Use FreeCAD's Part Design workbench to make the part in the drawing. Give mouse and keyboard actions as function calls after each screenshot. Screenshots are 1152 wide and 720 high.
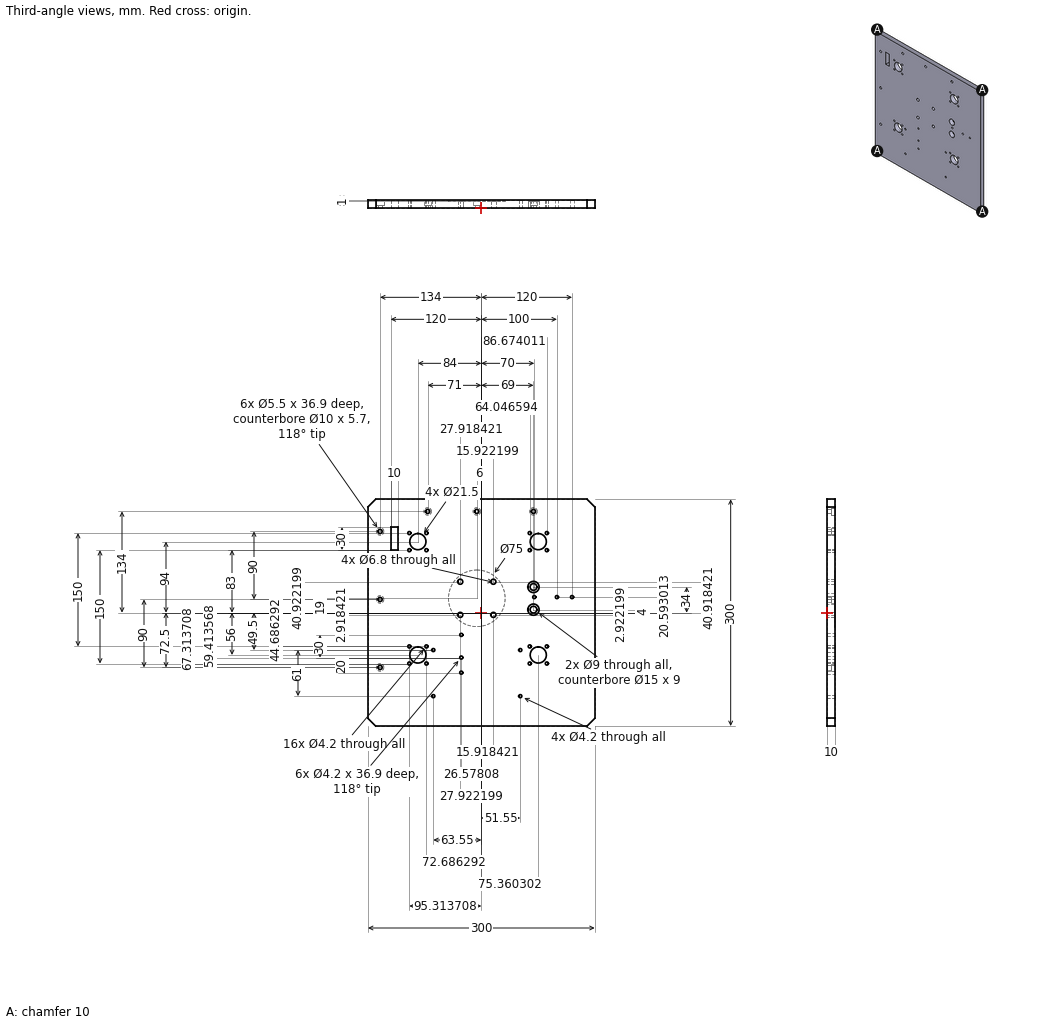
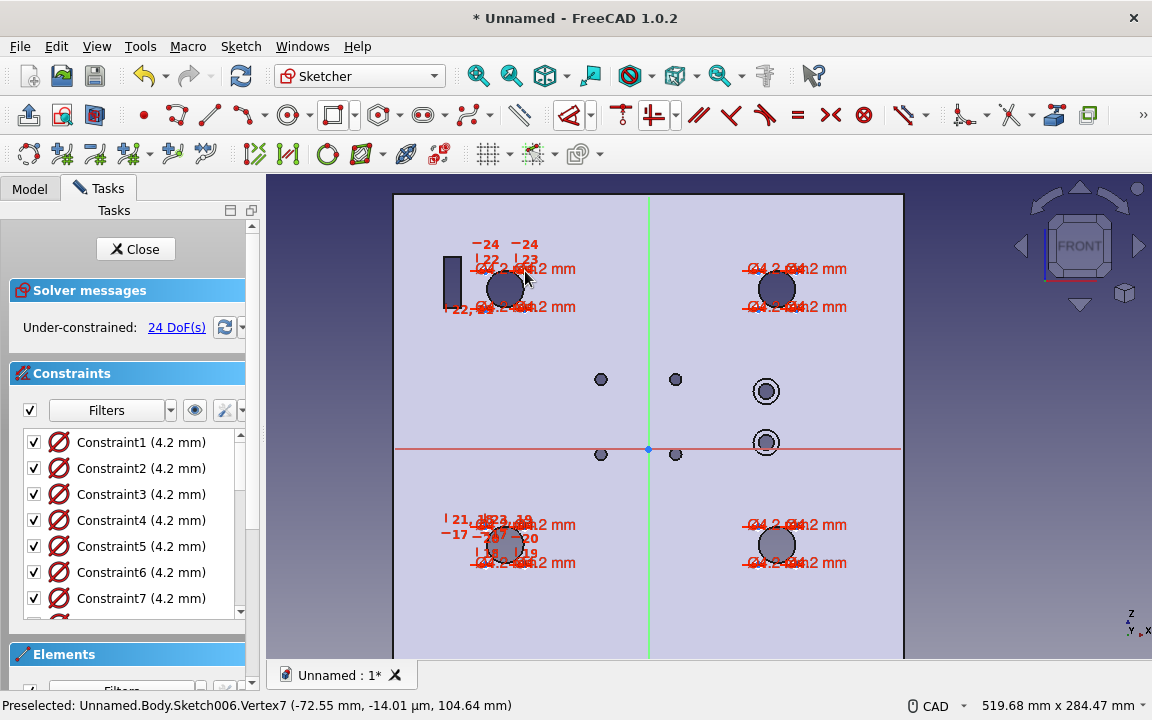
click(525, 309)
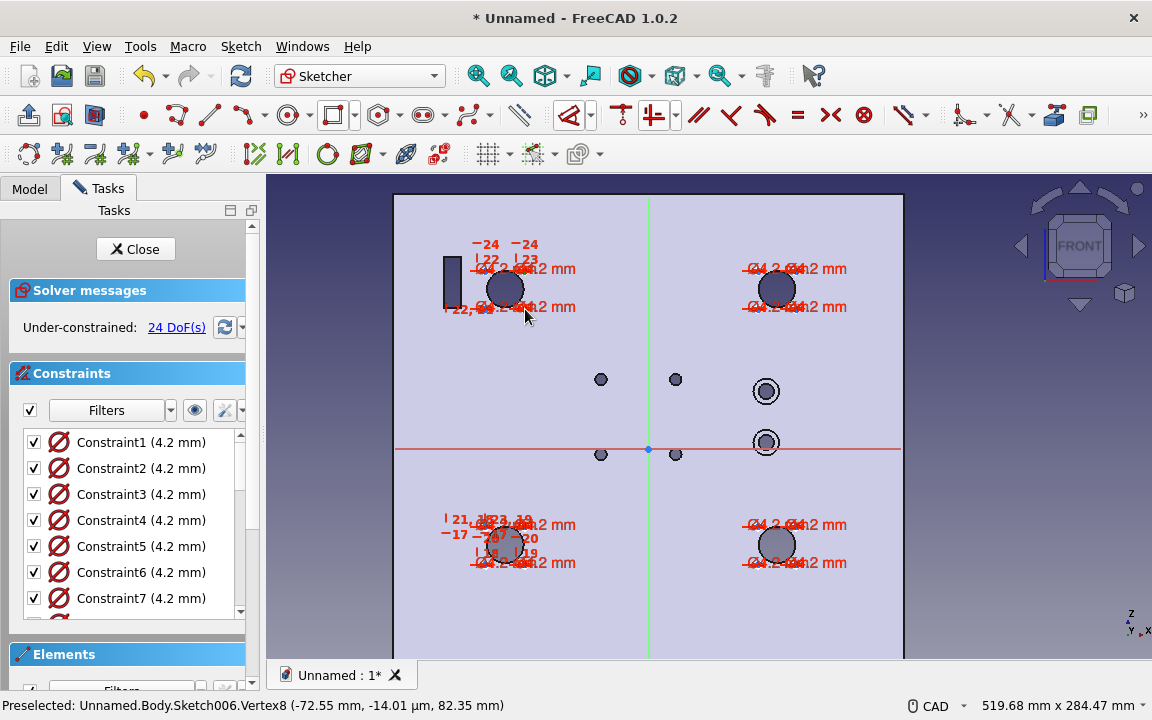
key(v)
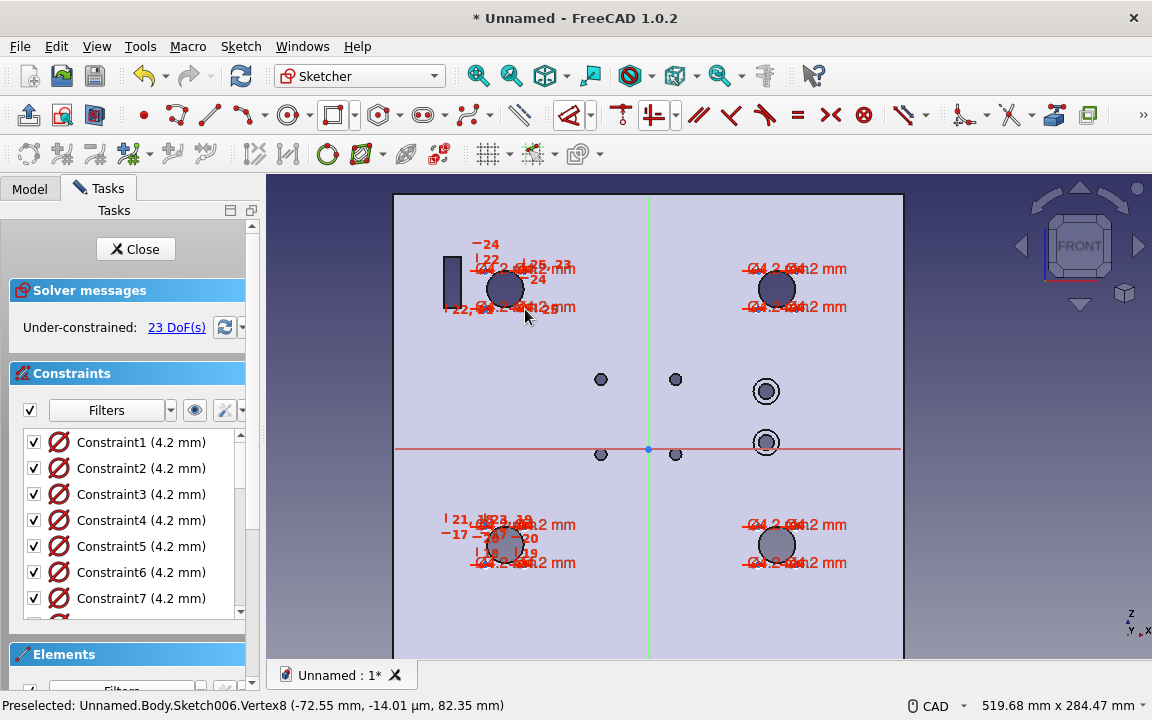
click(486, 309)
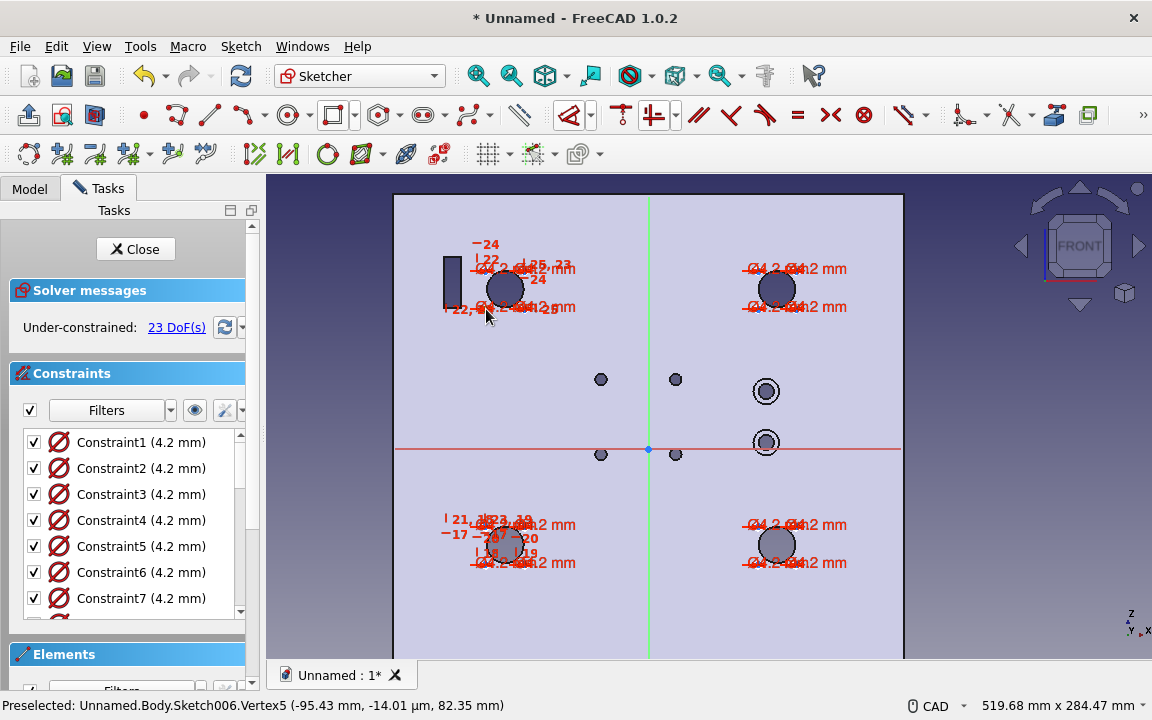
click(525, 309)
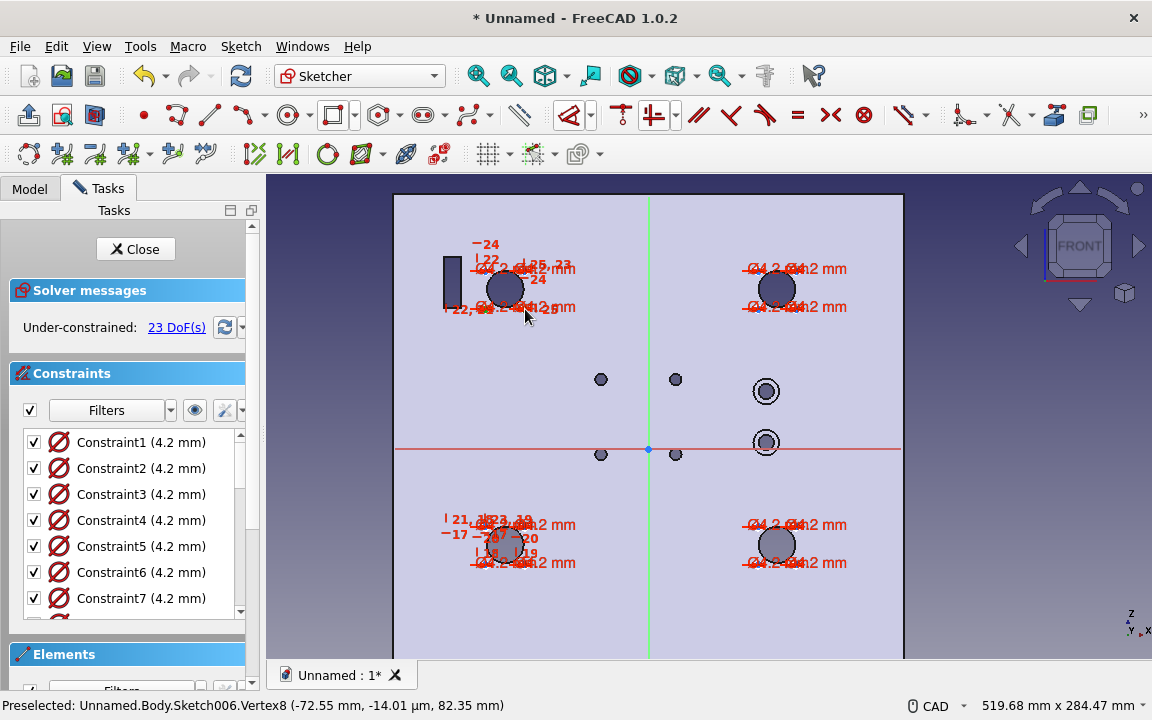
click(676, 116)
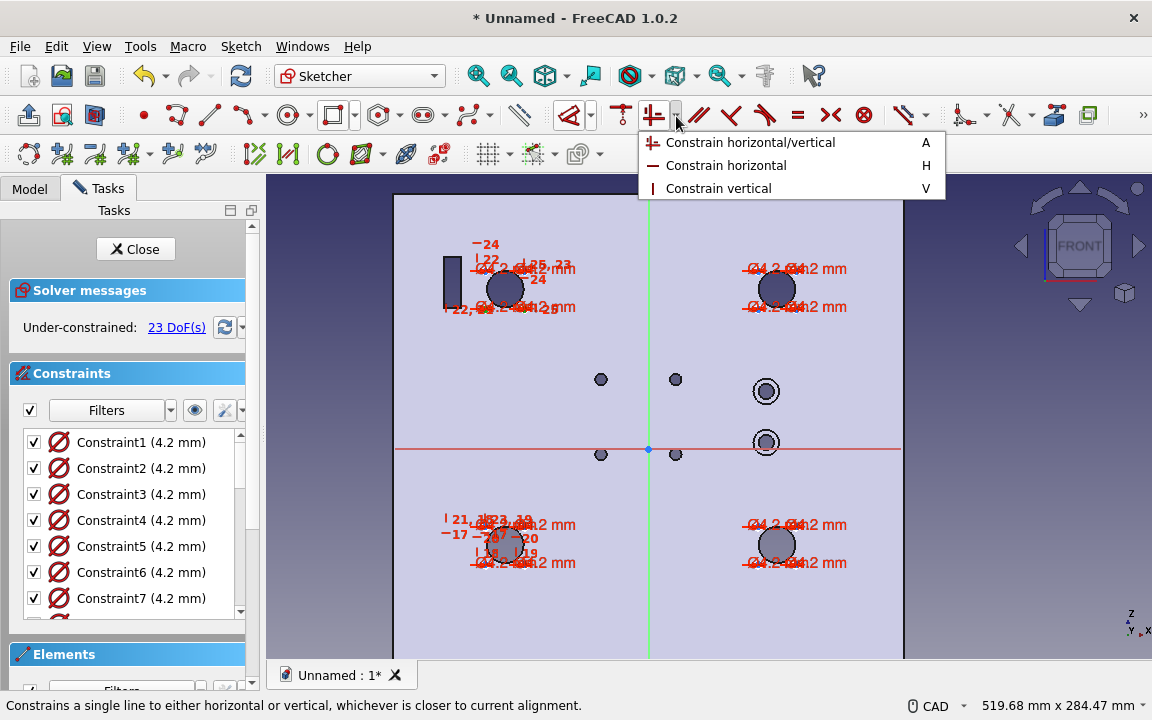
click(792, 166)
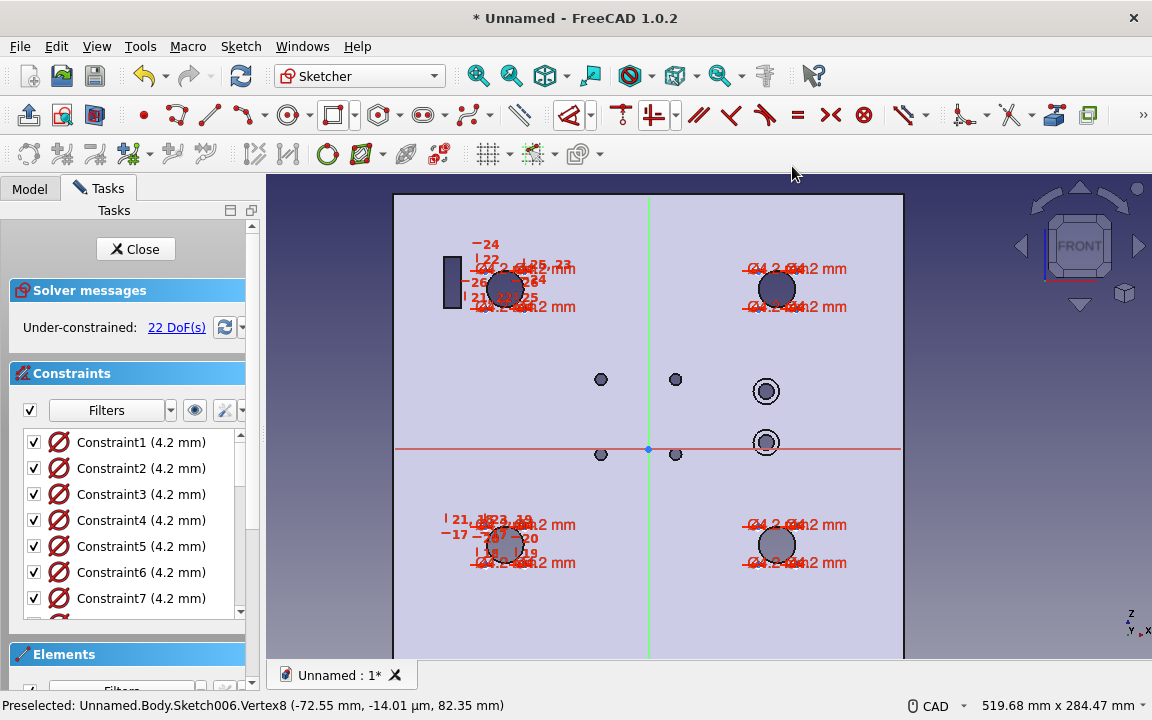
click(525, 309)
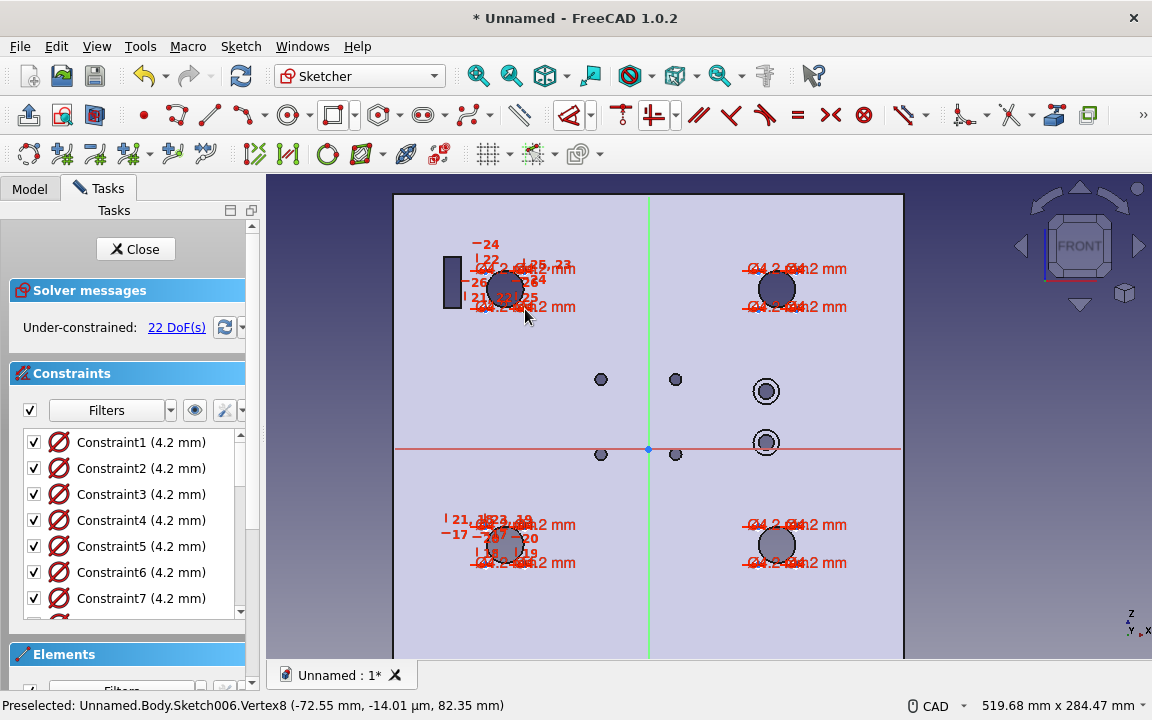
click(758, 309)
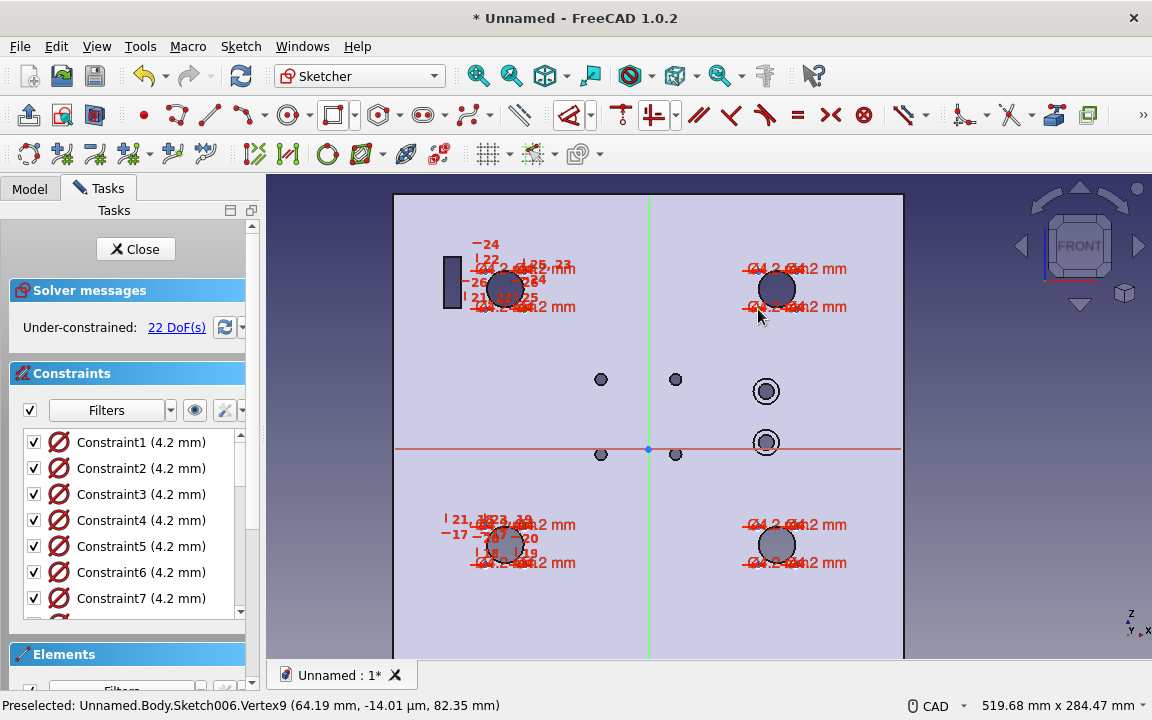
key(h)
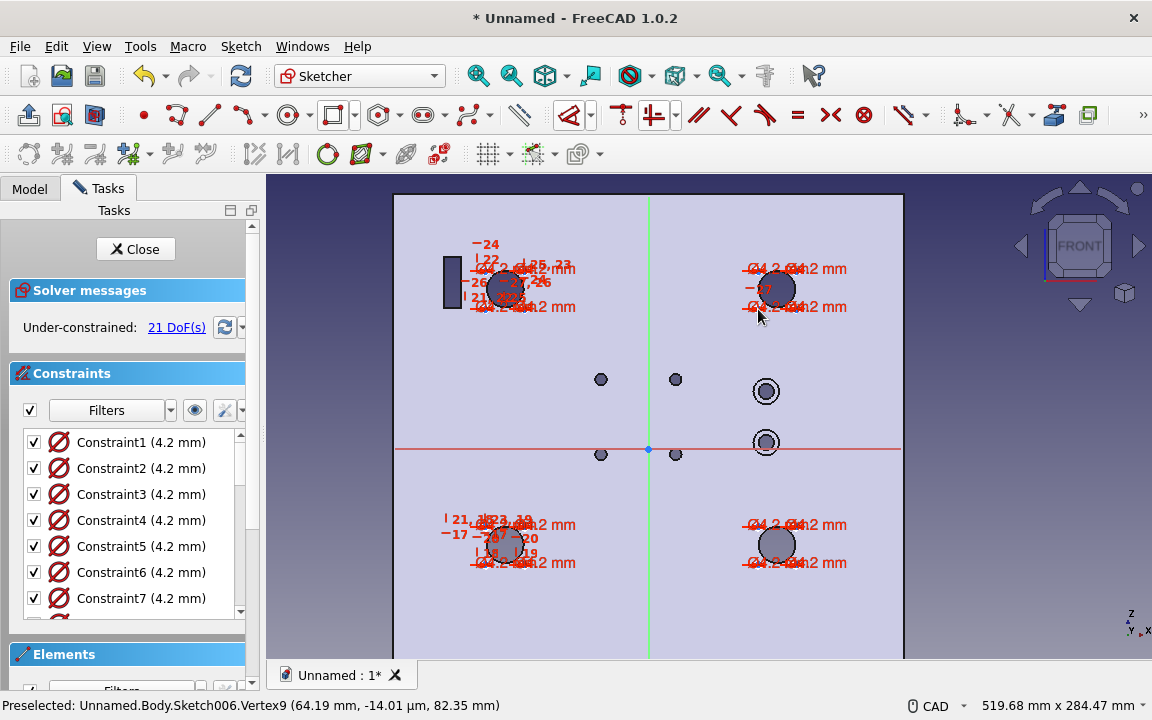
click(758, 309)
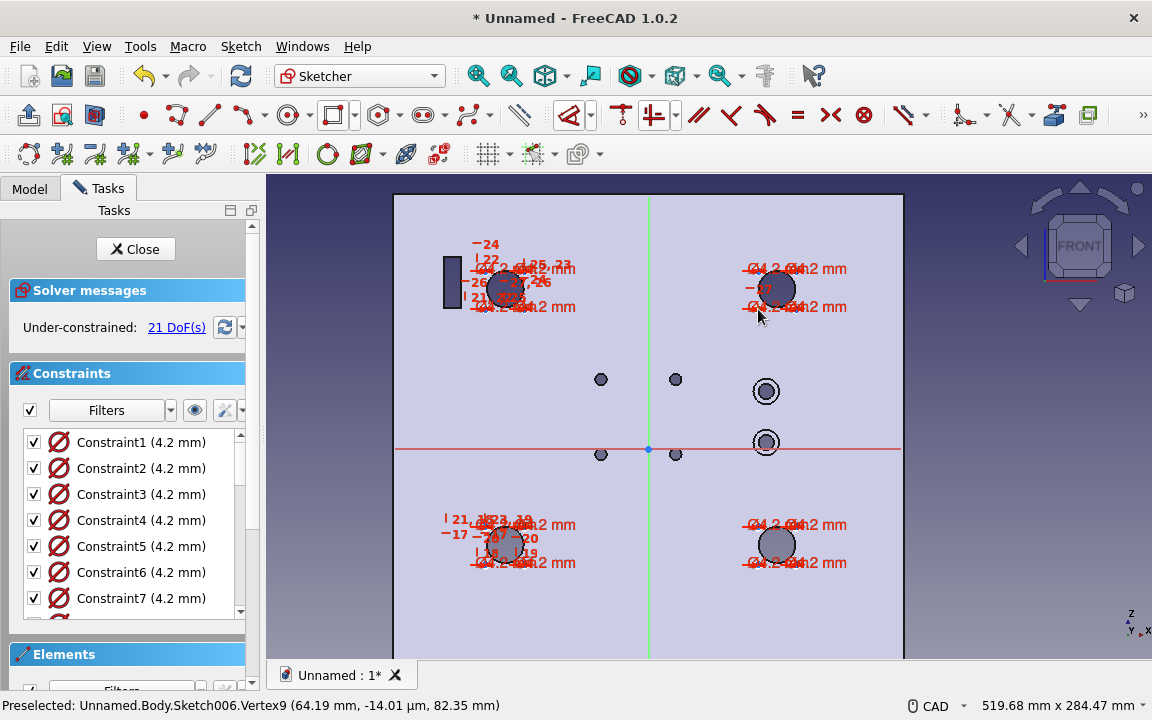
click(758, 271)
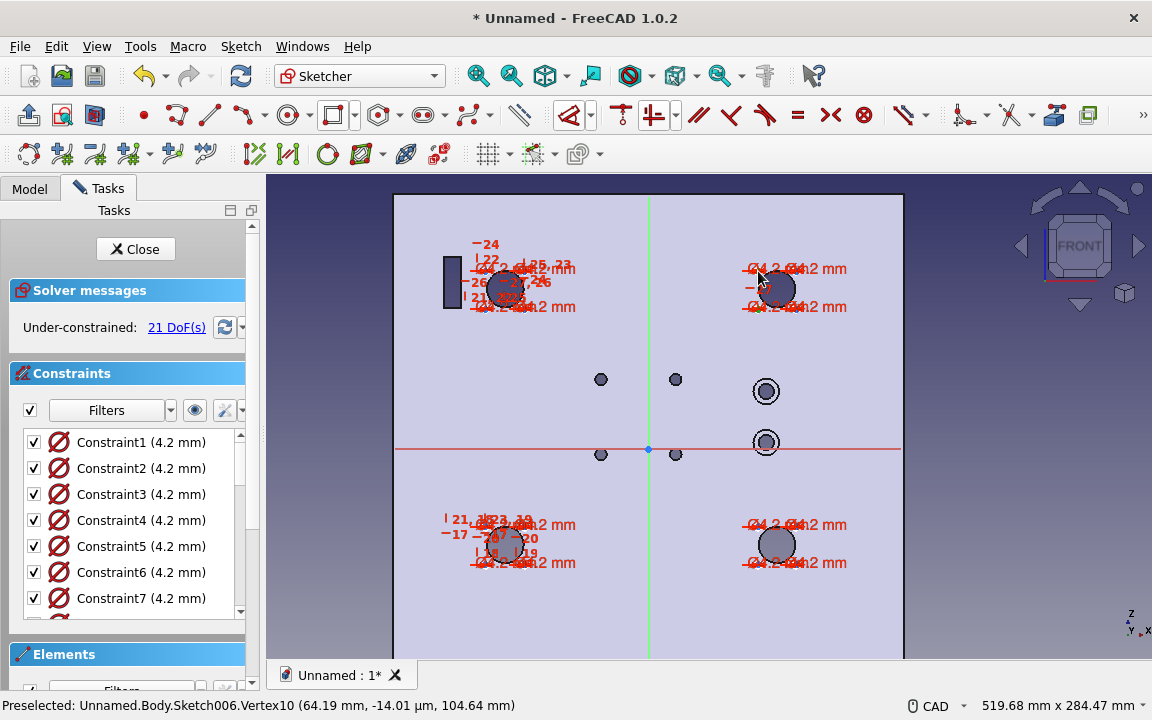
key(v)